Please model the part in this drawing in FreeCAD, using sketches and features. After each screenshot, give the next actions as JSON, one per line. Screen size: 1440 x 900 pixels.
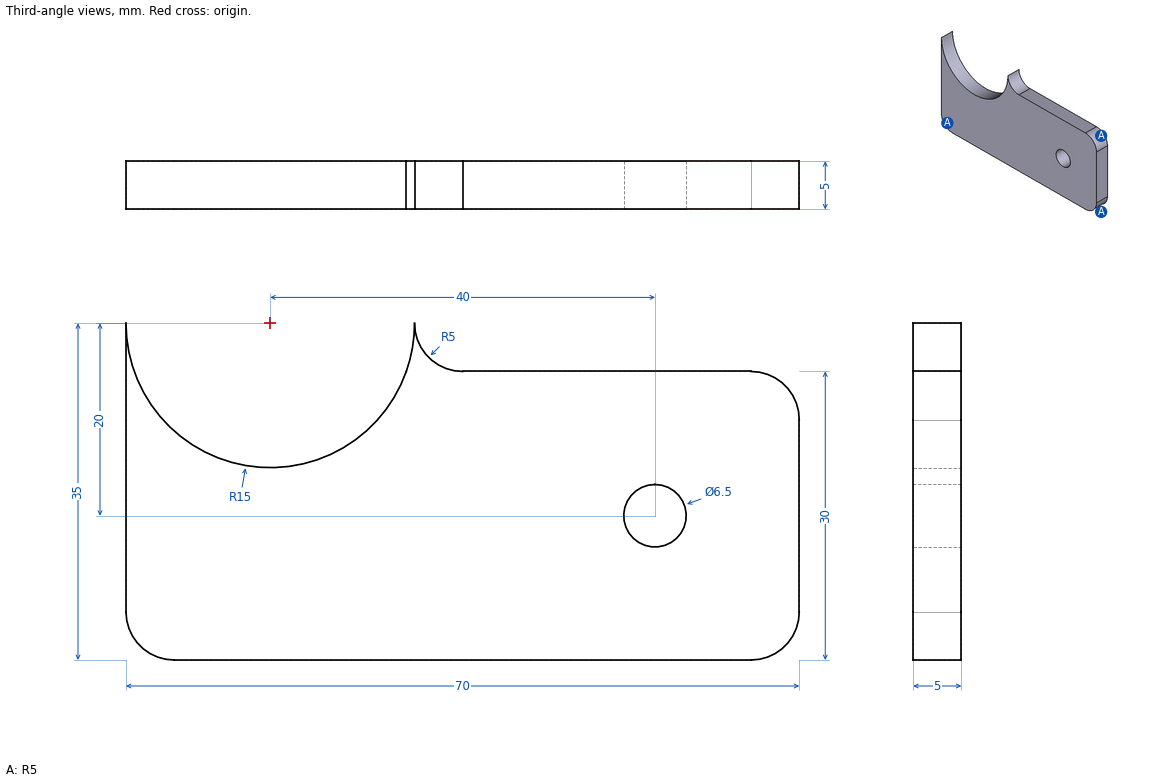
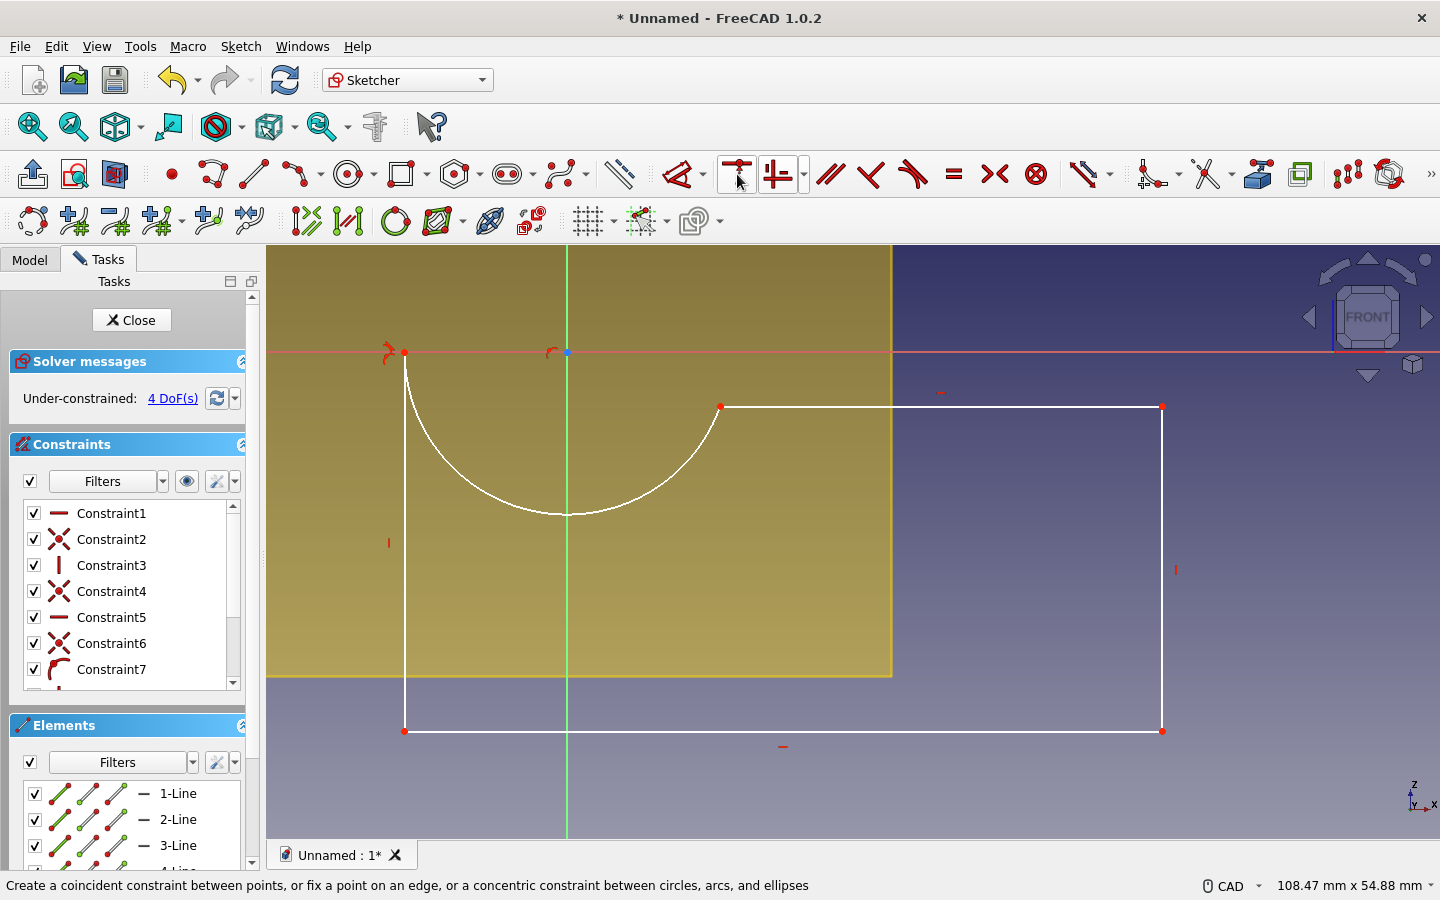
{"action": "left_click", "coordinate": [676, 174]}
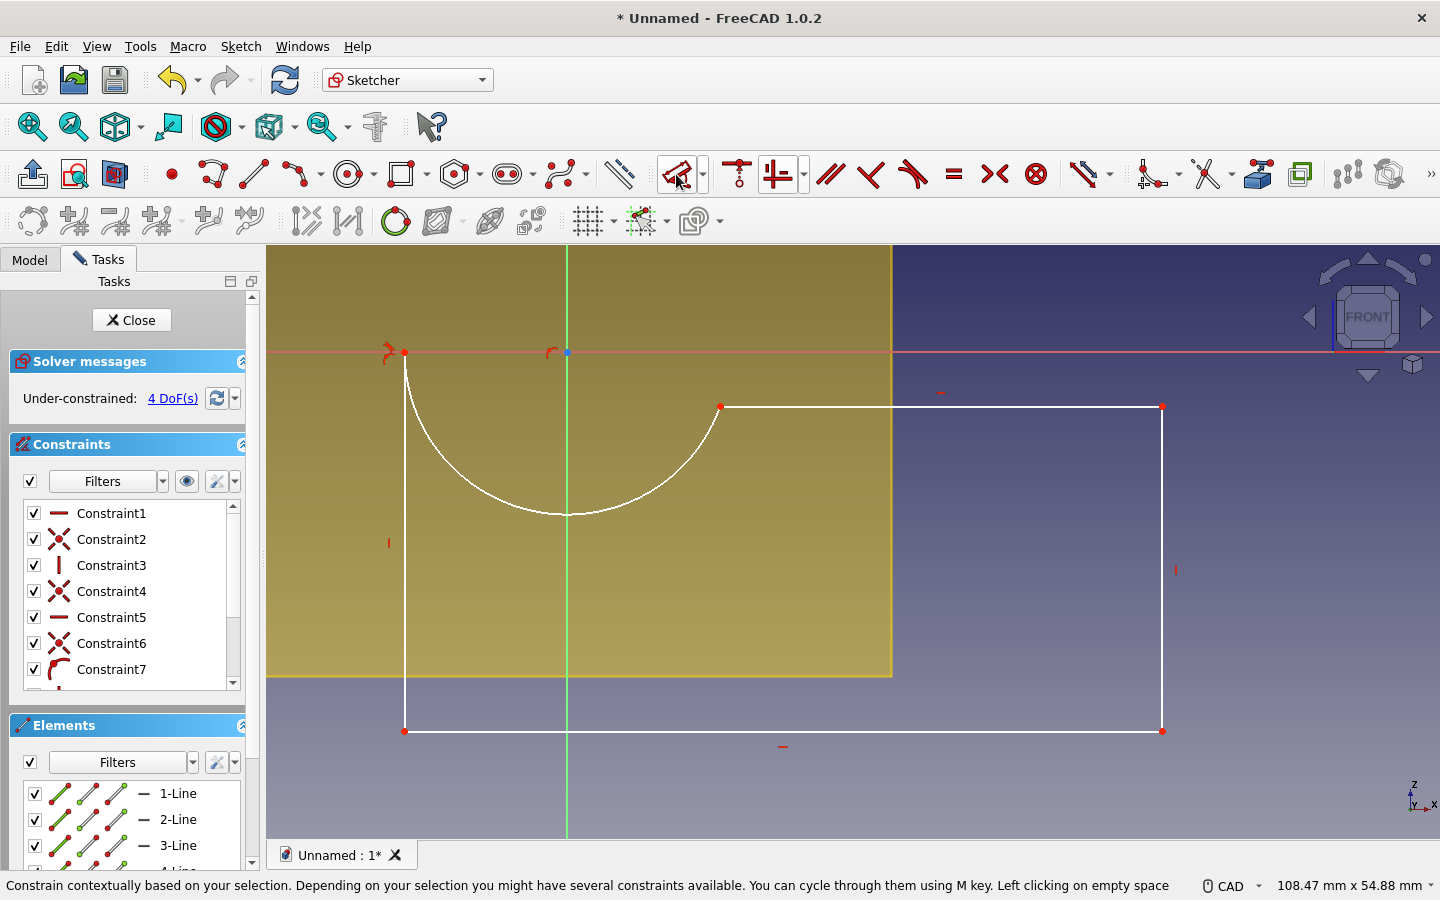
{"action": "left_click", "coordinate": [459, 473]}
{"action": "left_click", "coordinate": [438, 497]}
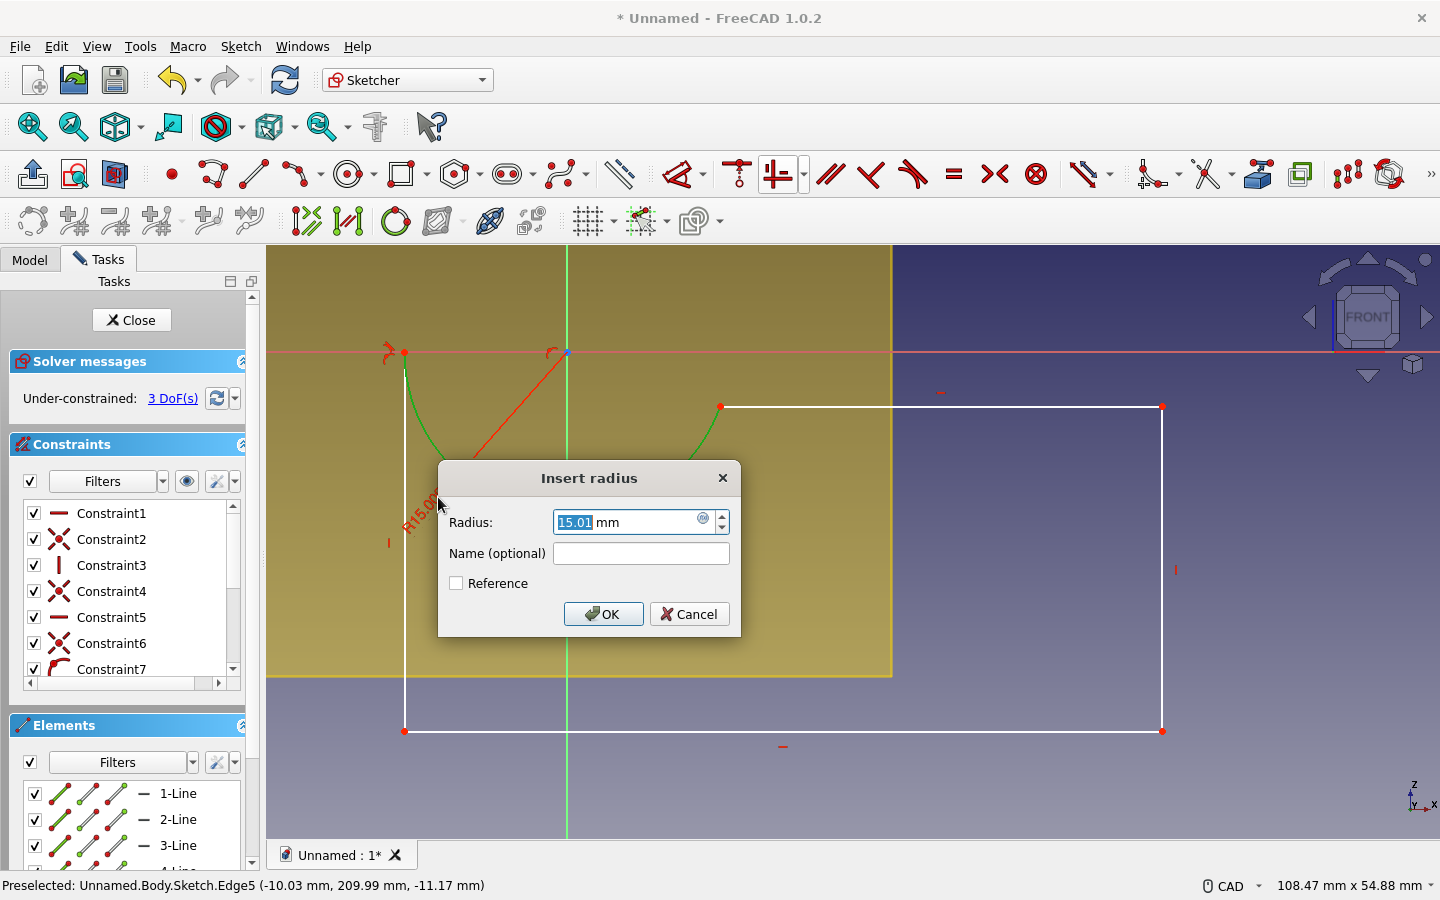
{"action": "type", "text": "15"}
{"action": "key", "text": "Return"}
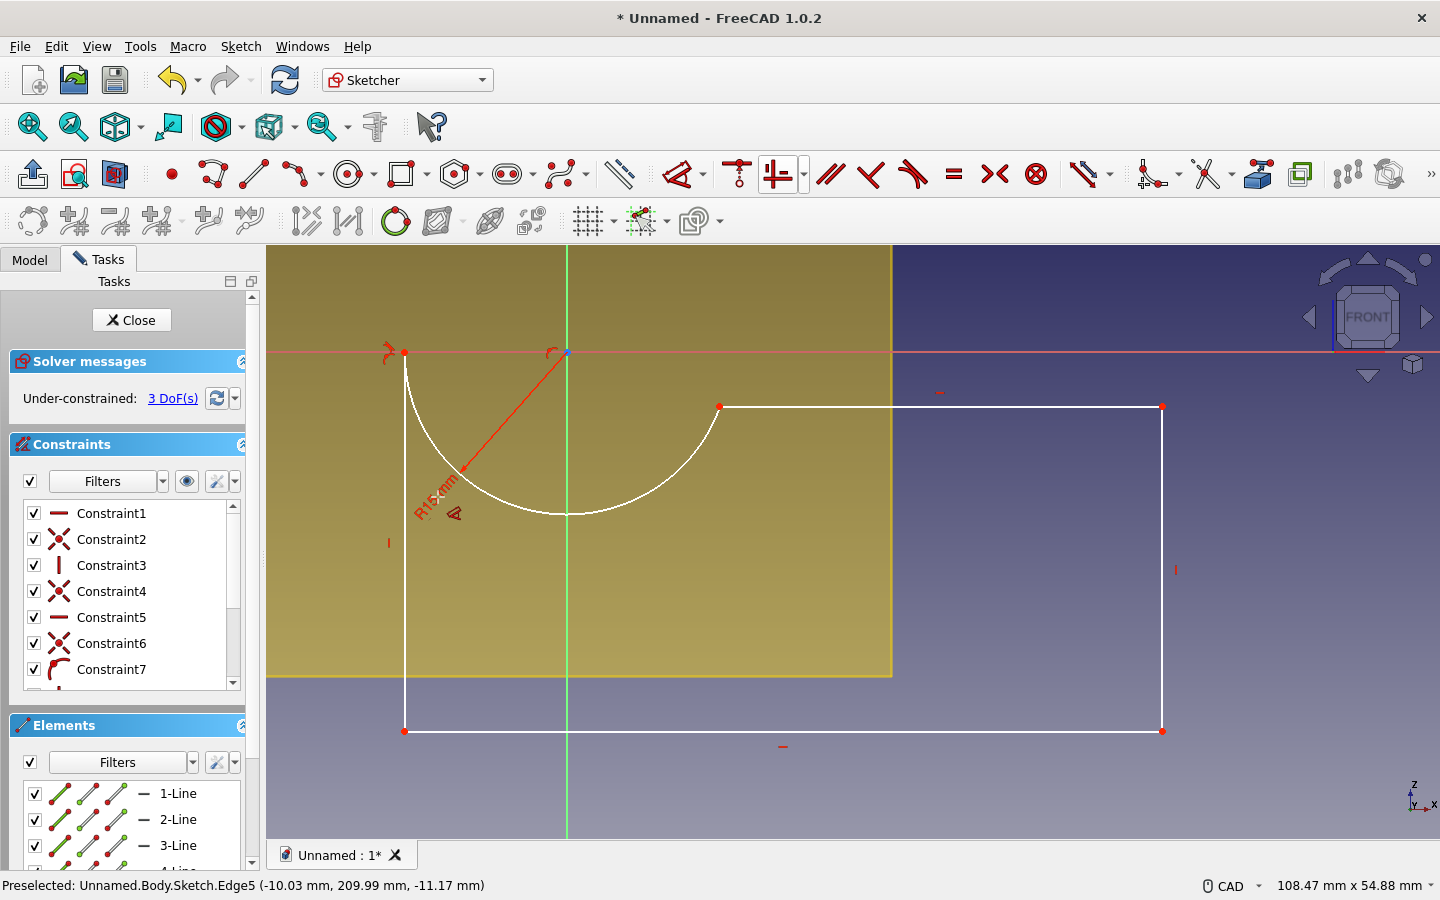
{"action": "left_click", "coordinate": [1162, 504]}
{"action": "left_click", "coordinate": [1196, 569]}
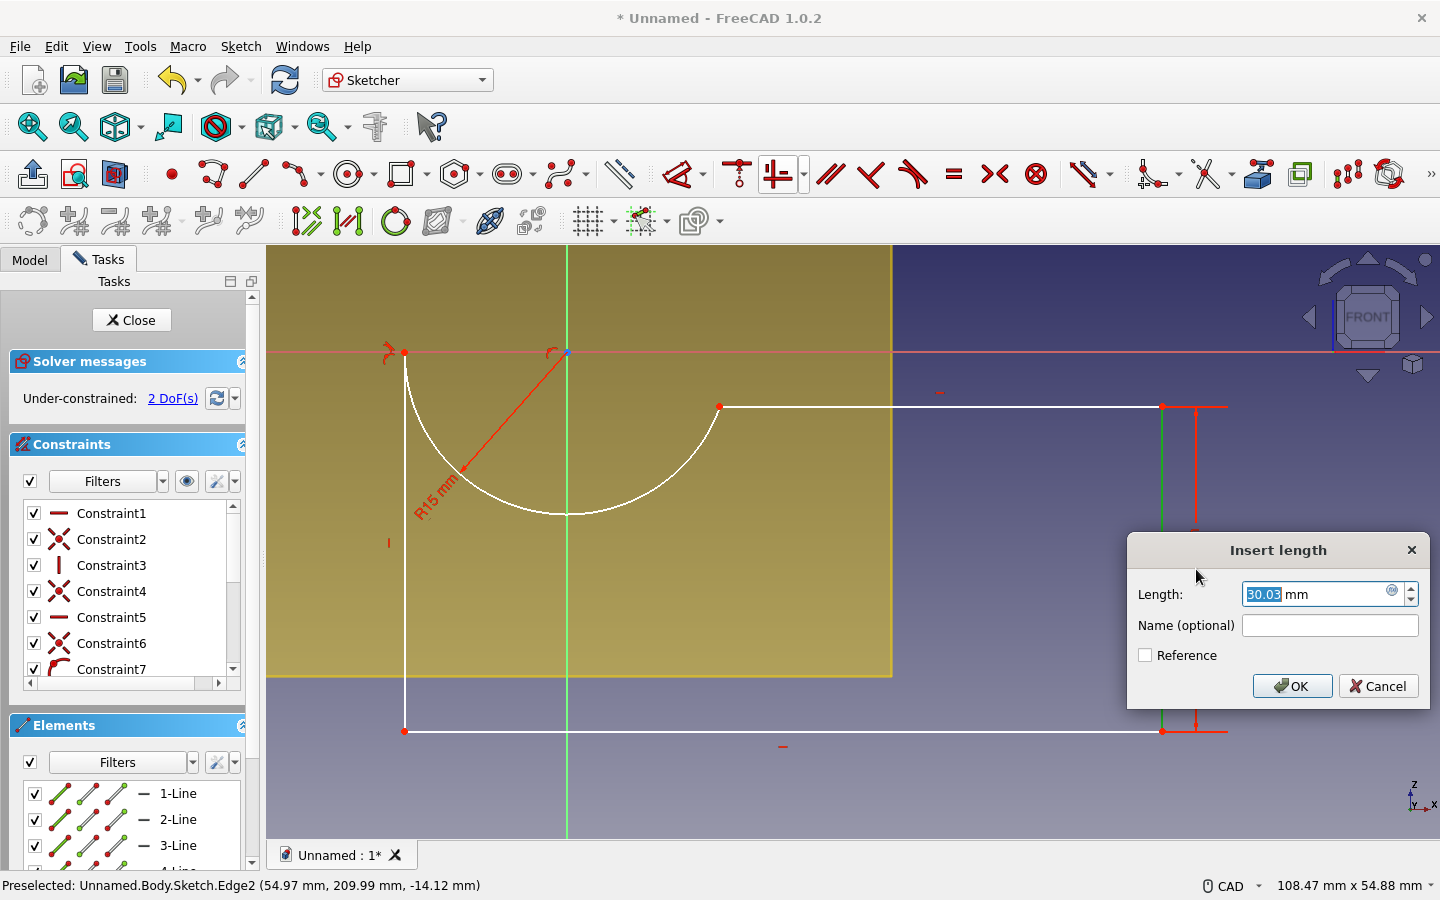
{"action": "type", "text": "30"}
{"action": "key", "text": "Return"}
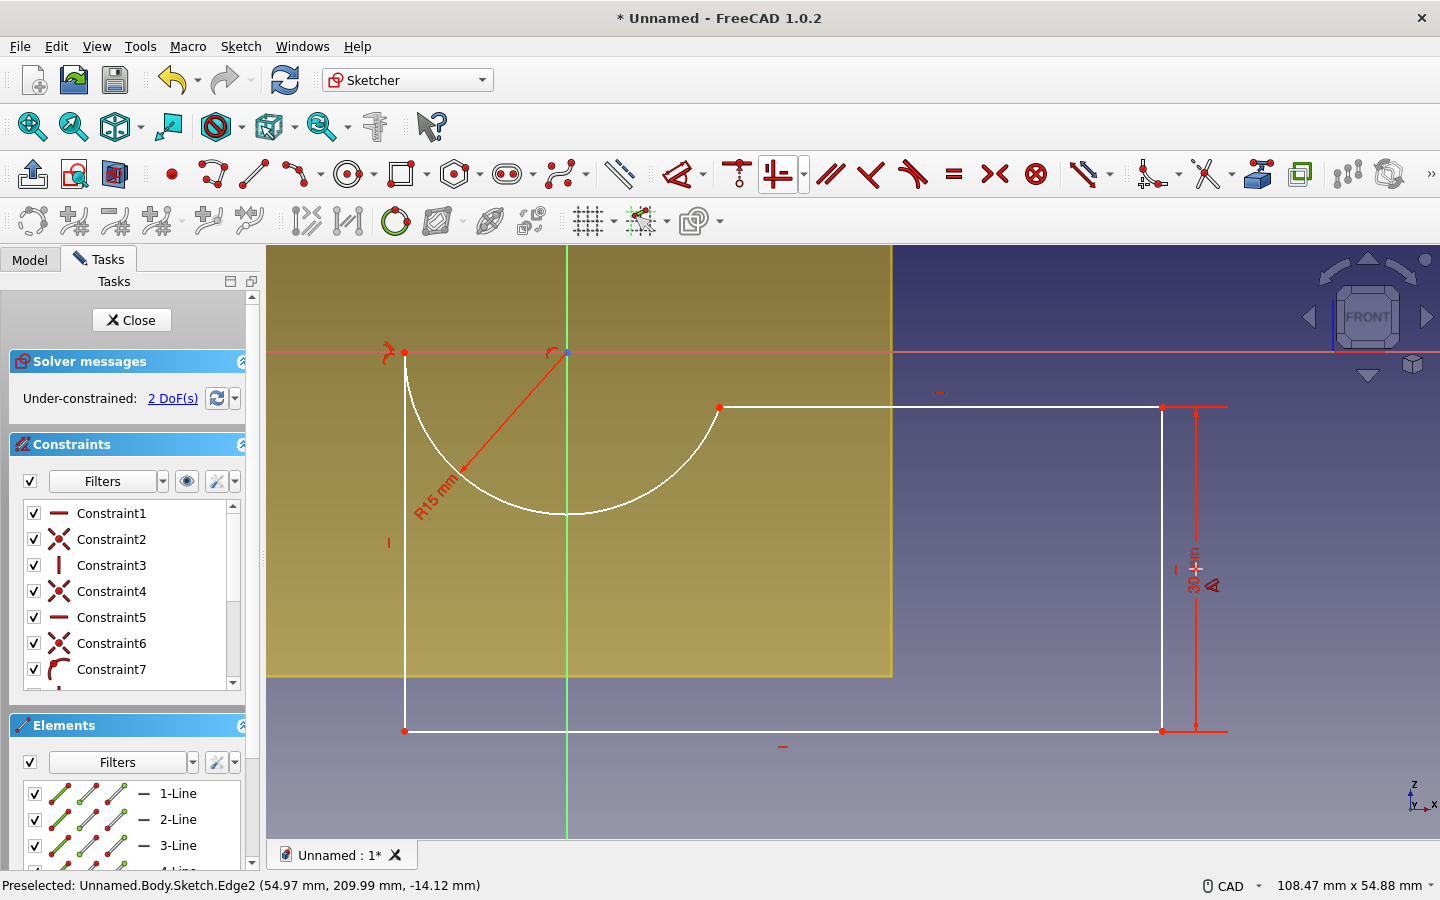
{"action": "left_click", "coordinate": [935, 732]}
{"action": "left_click", "coordinate": [783, 766]}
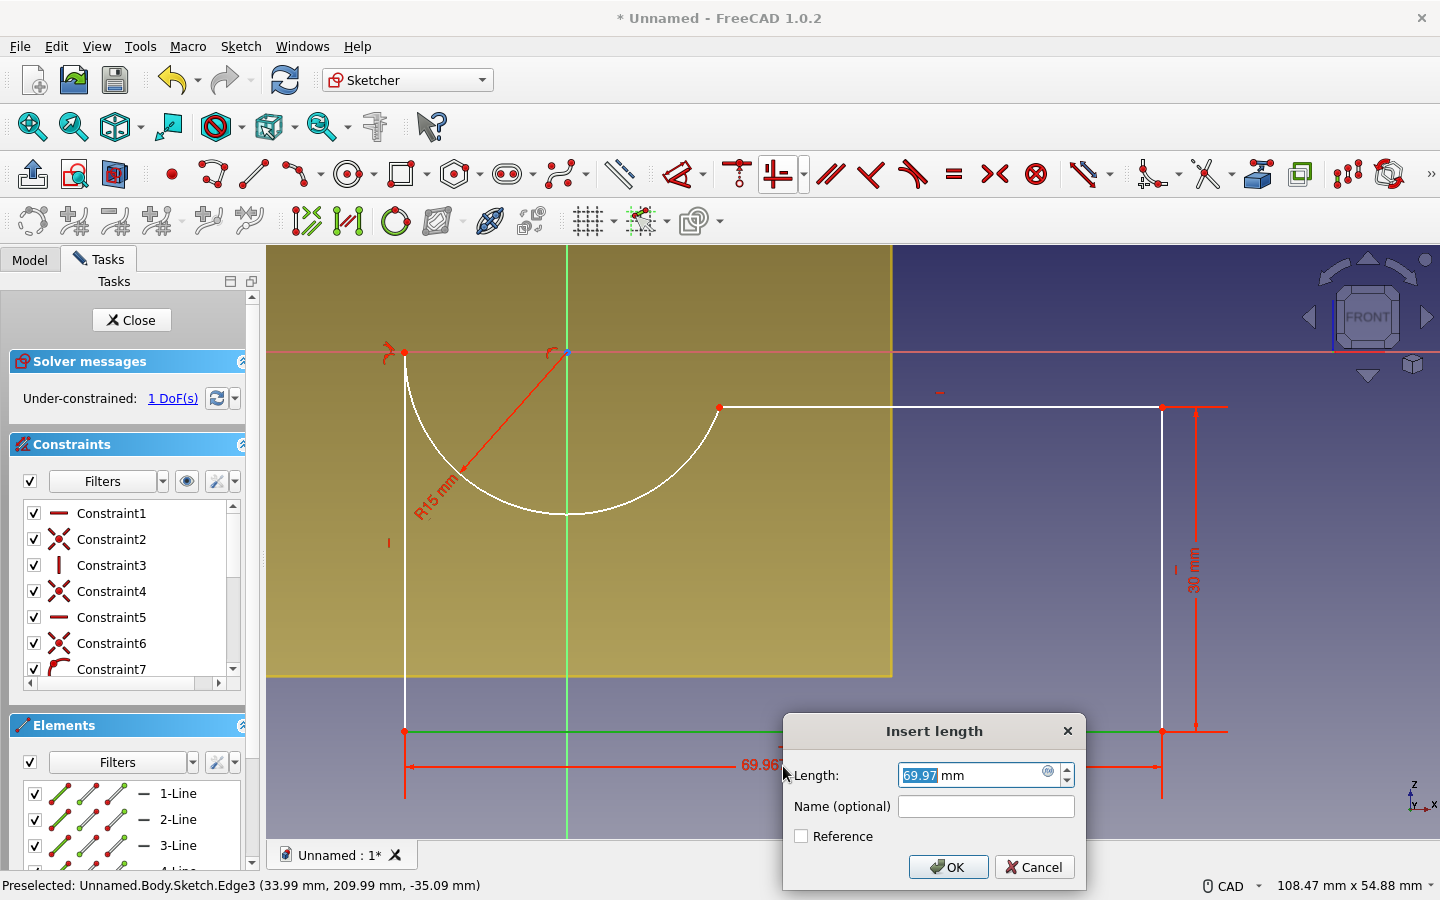
{"action": "type", "text": "70"}
{"action": "key", "text": "Return"}